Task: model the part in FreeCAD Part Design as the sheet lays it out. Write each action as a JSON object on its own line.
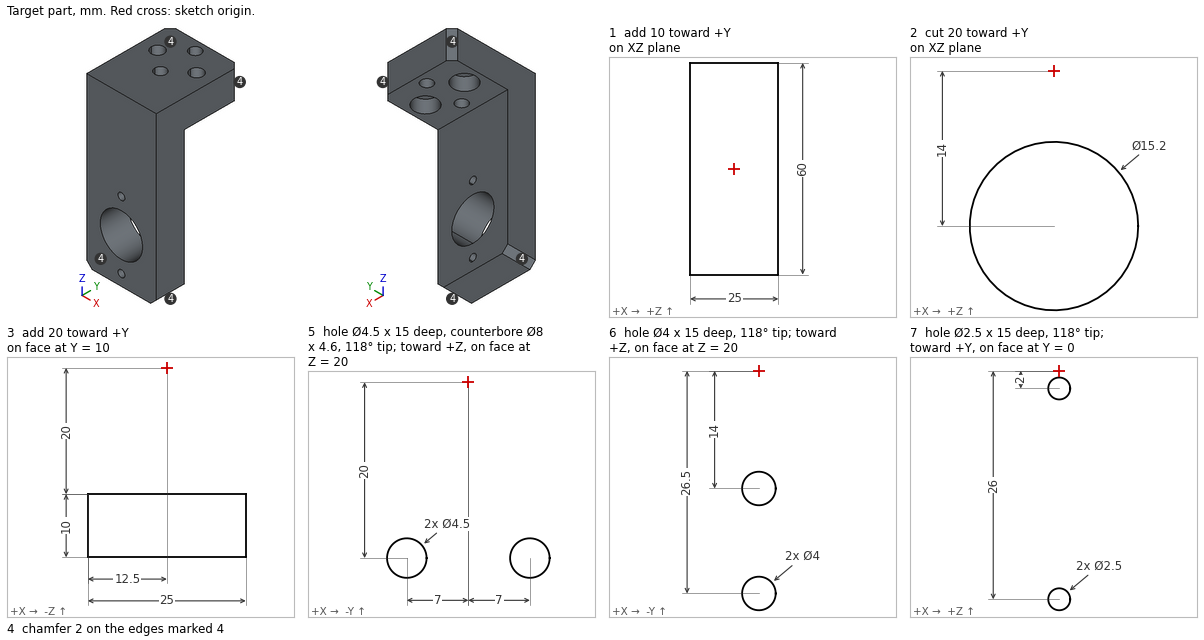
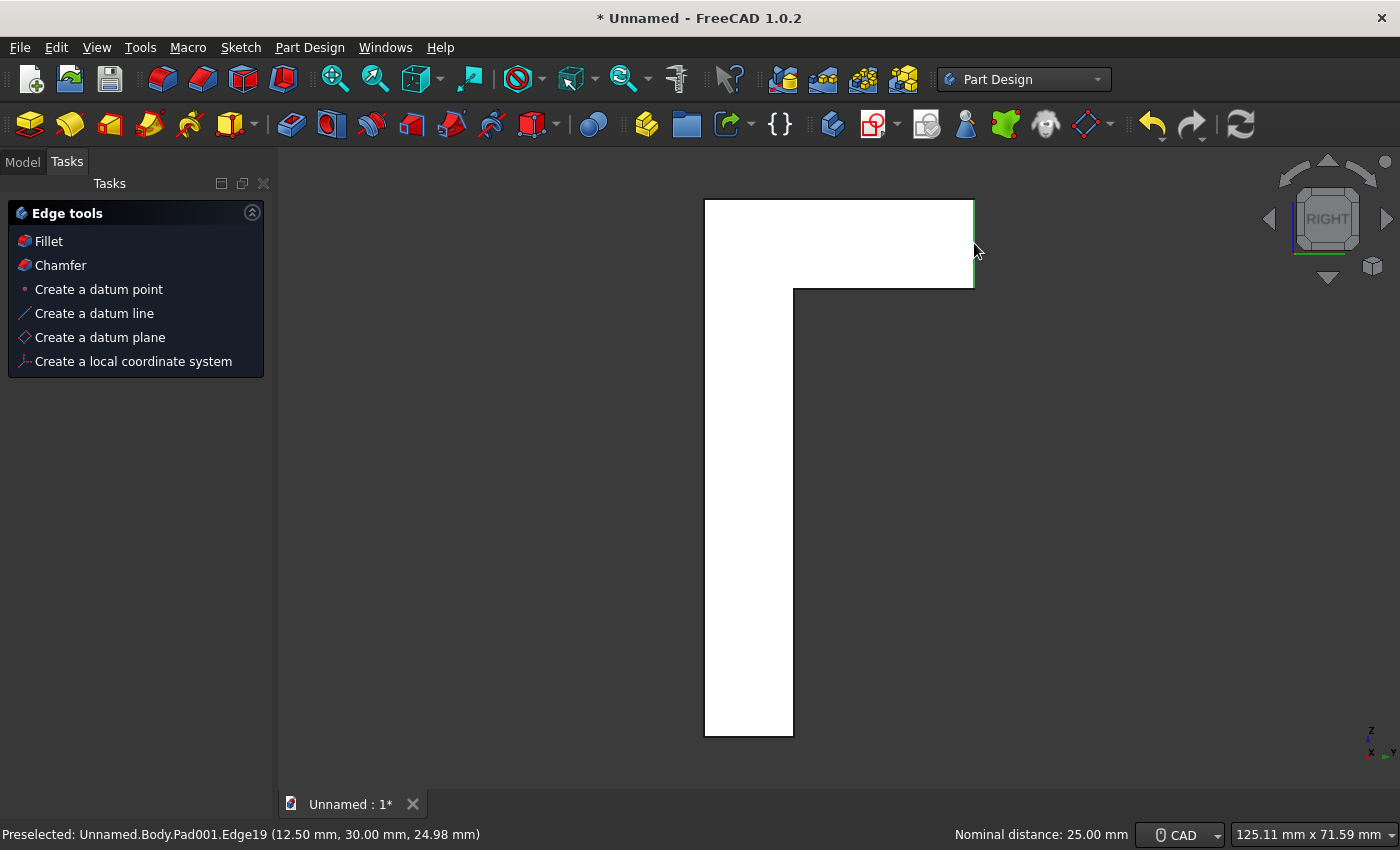
{"action": "left_click", "coordinate": [749, 736], "text": "ctrl"}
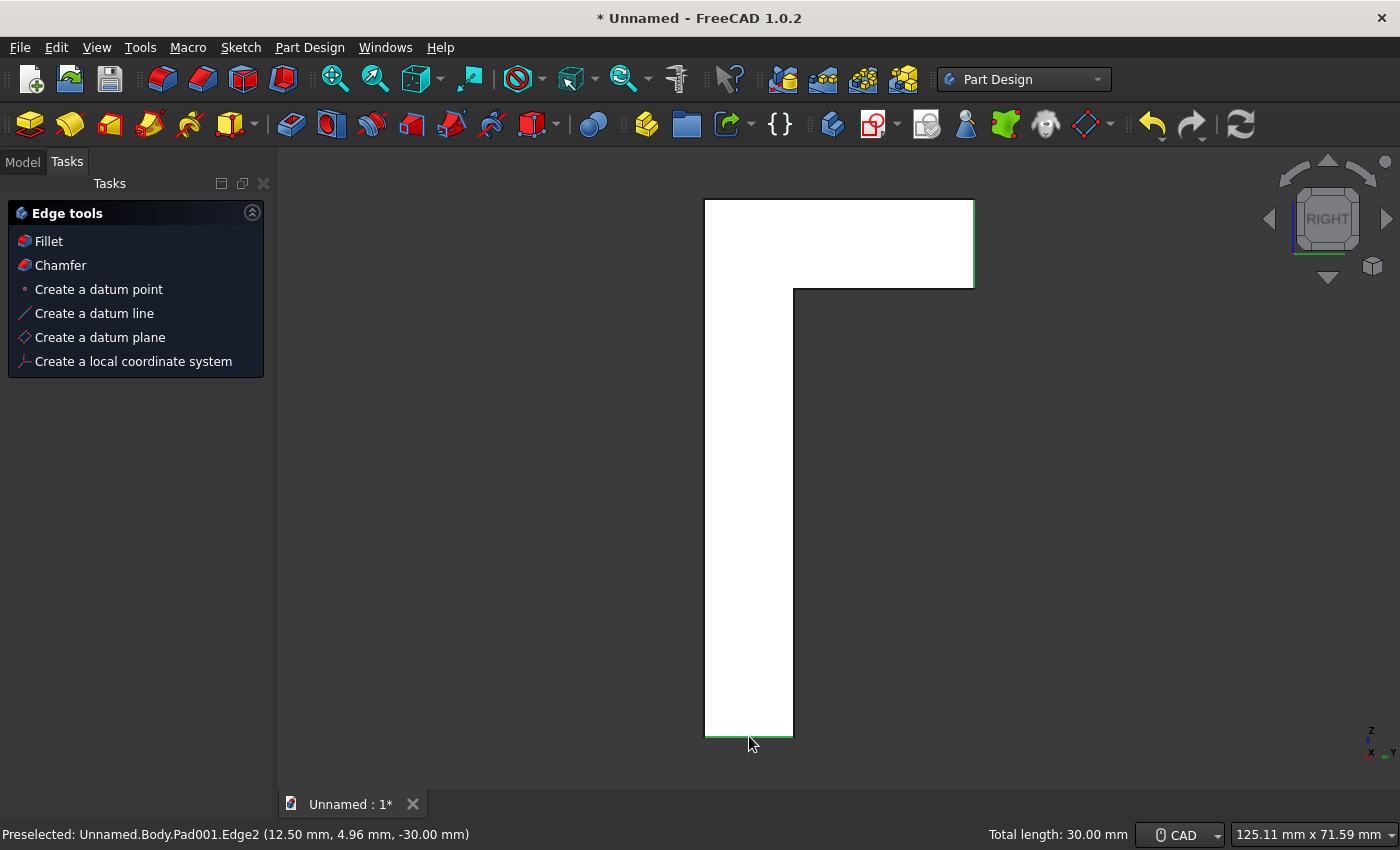
{"action": "key", "text": "5"}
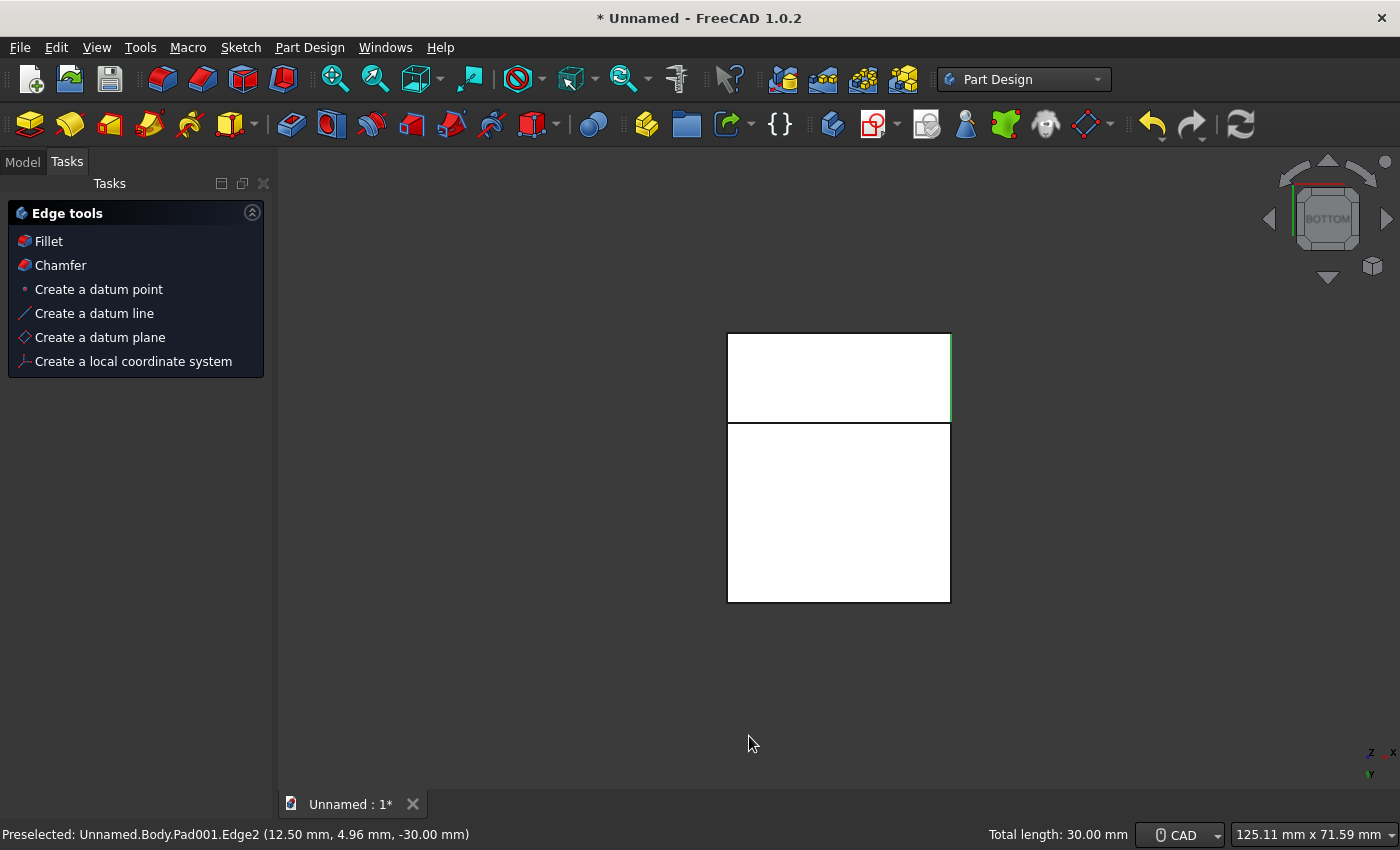
{"action": "key", "text": "v f"}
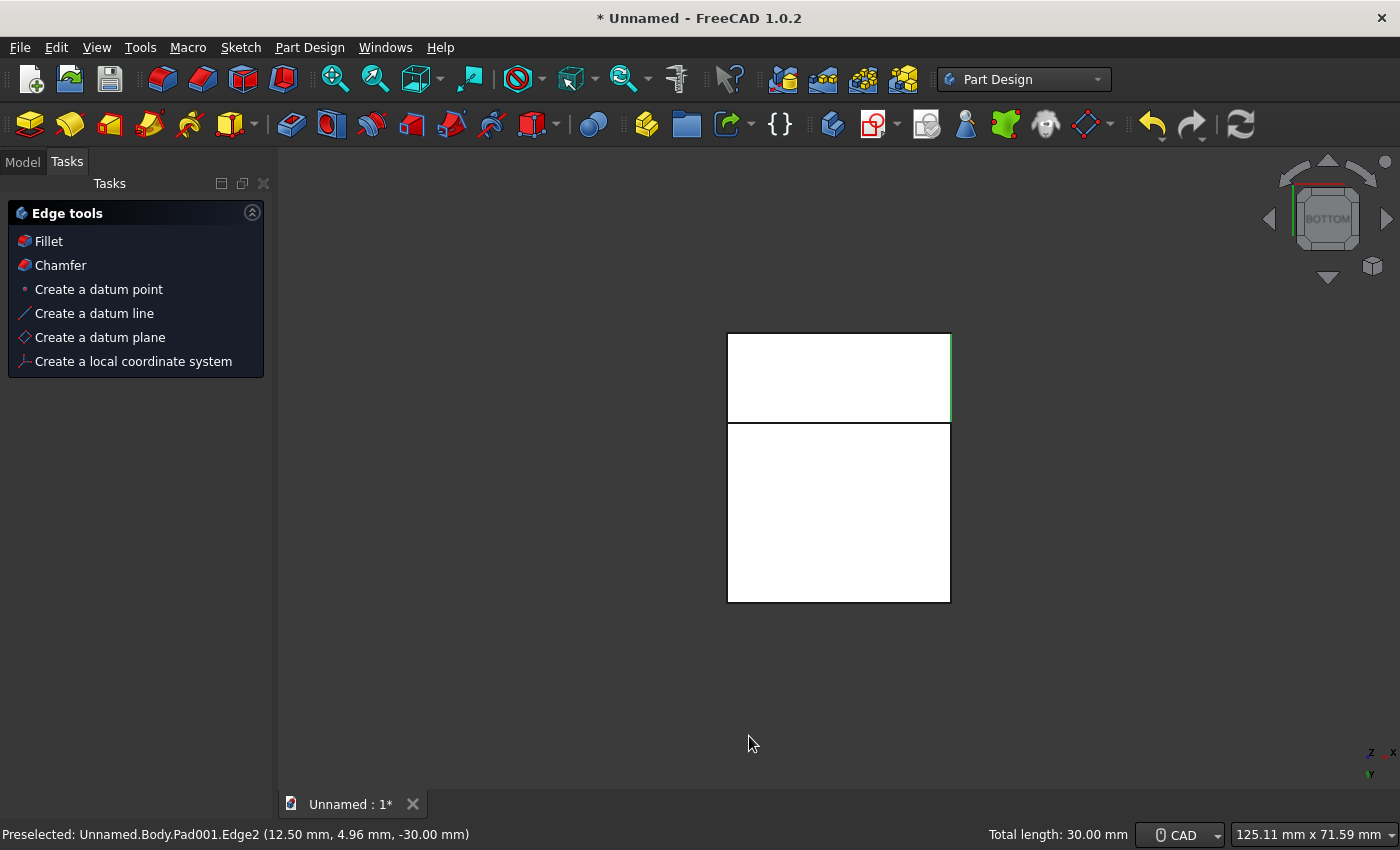
{"action": "left_click", "coordinate": [727, 377], "text": "ctrl"}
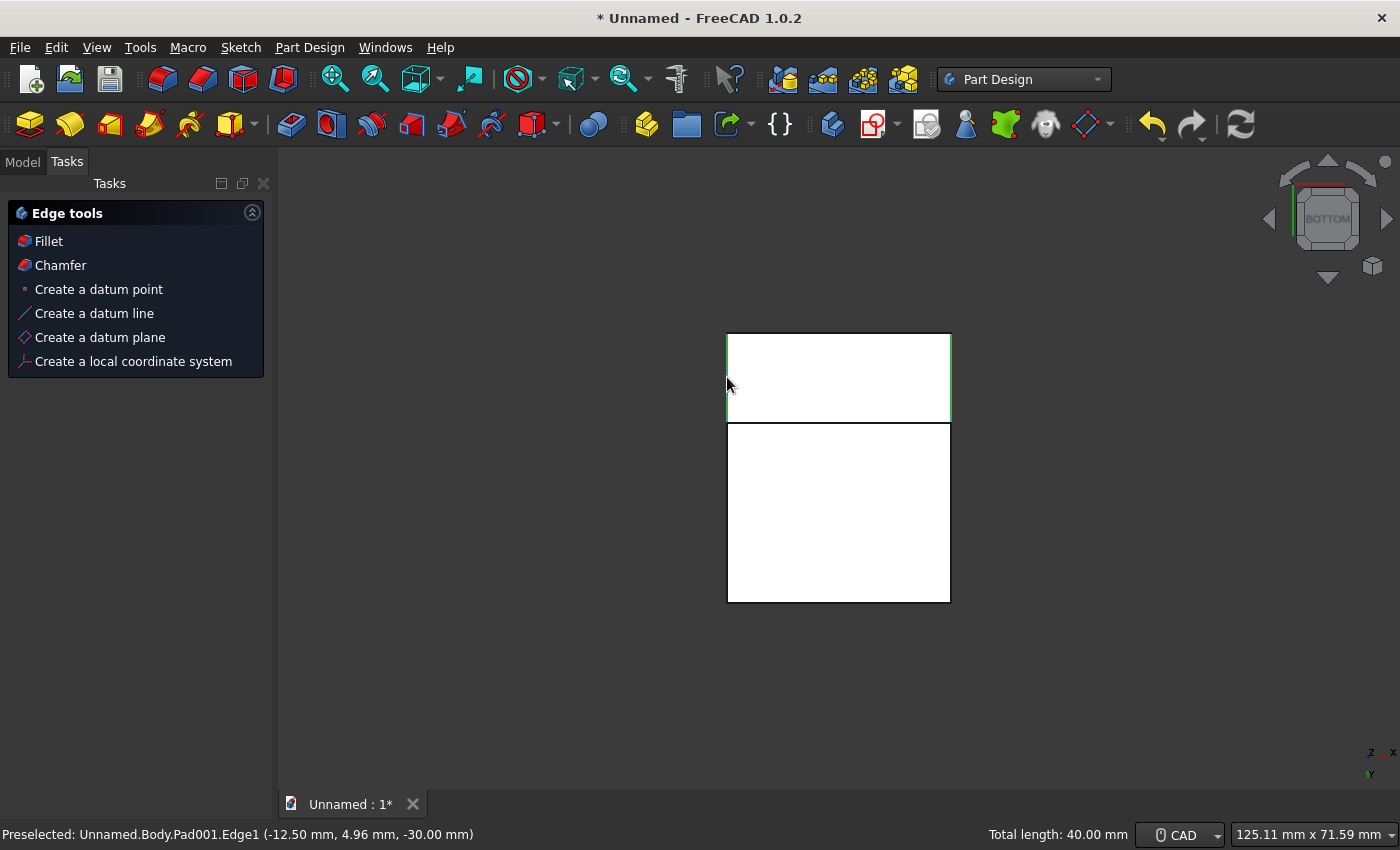
{"action": "left_click", "coordinate": [204, 80]}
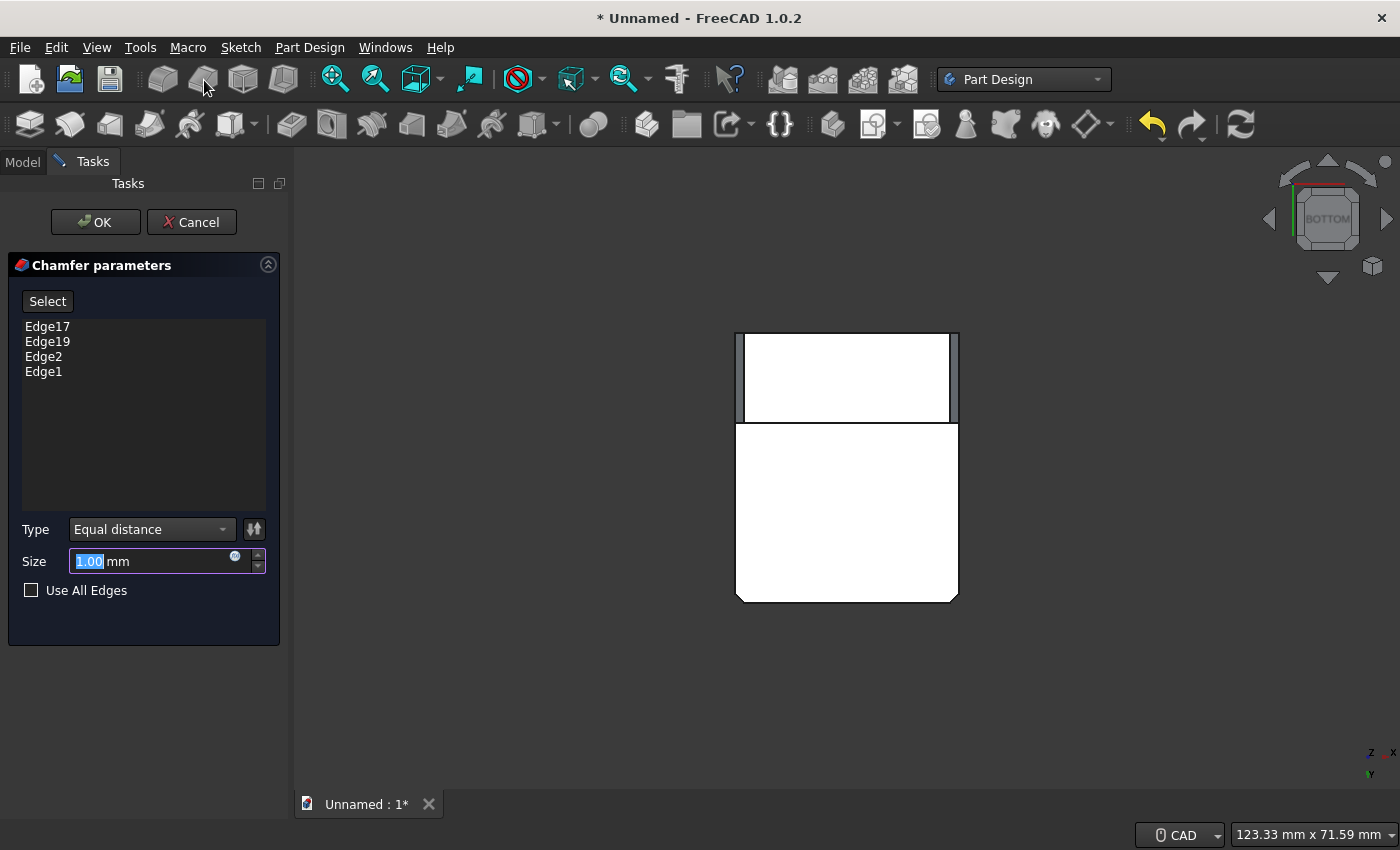
{"action": "type", "text": "2"}
{"action": "key", "text": "Tab"}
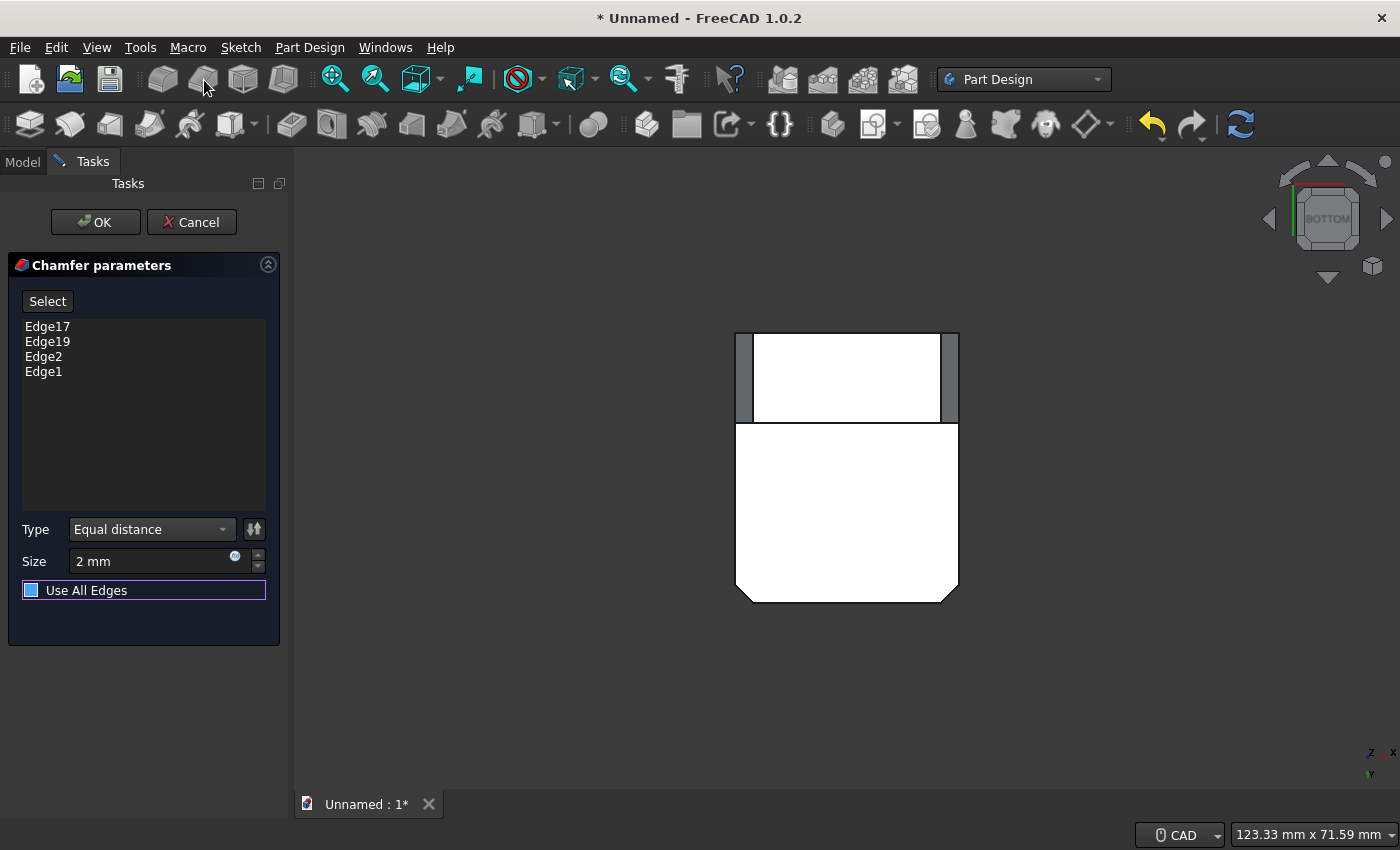
{"action": "left_click", "coordinate": [96, 222]}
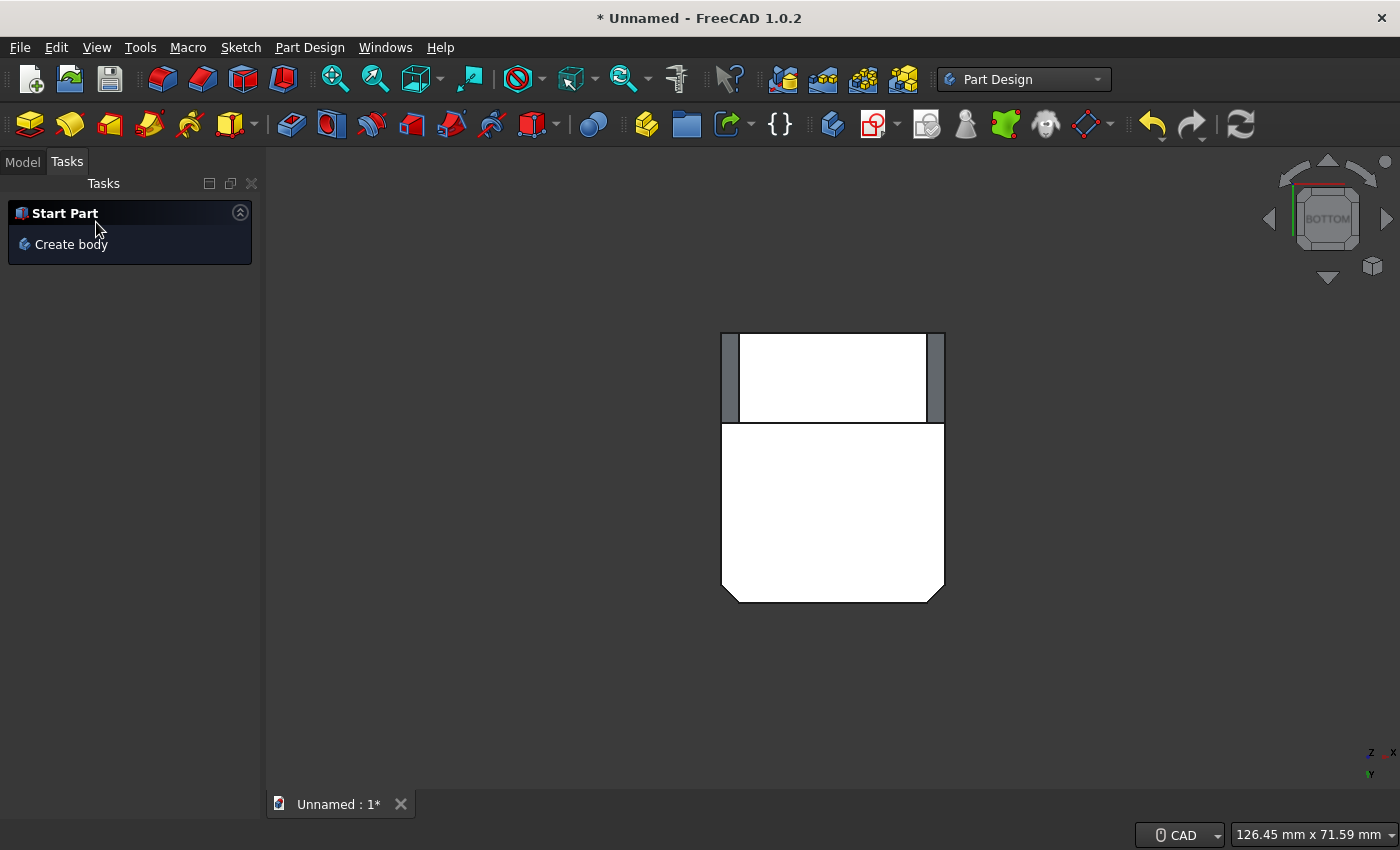
{"action": "key", "text": "v f"}